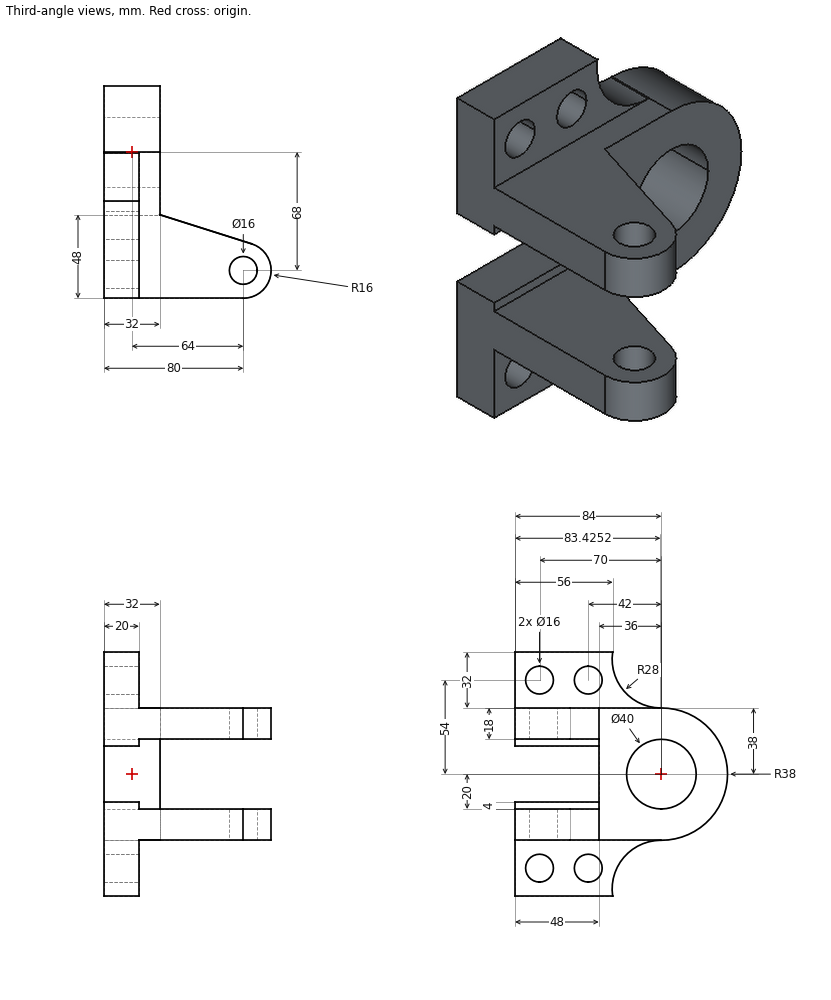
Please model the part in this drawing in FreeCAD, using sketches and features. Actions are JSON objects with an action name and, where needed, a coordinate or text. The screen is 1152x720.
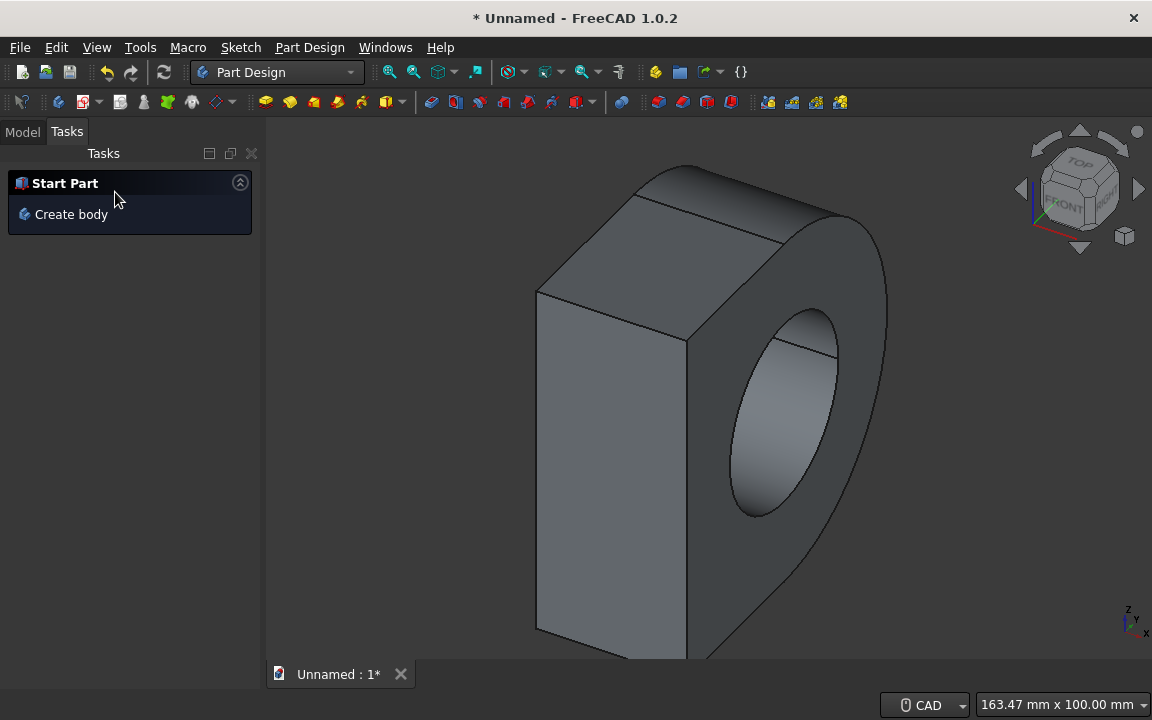
{"action": "left_click", "coordinate": [390, 72]}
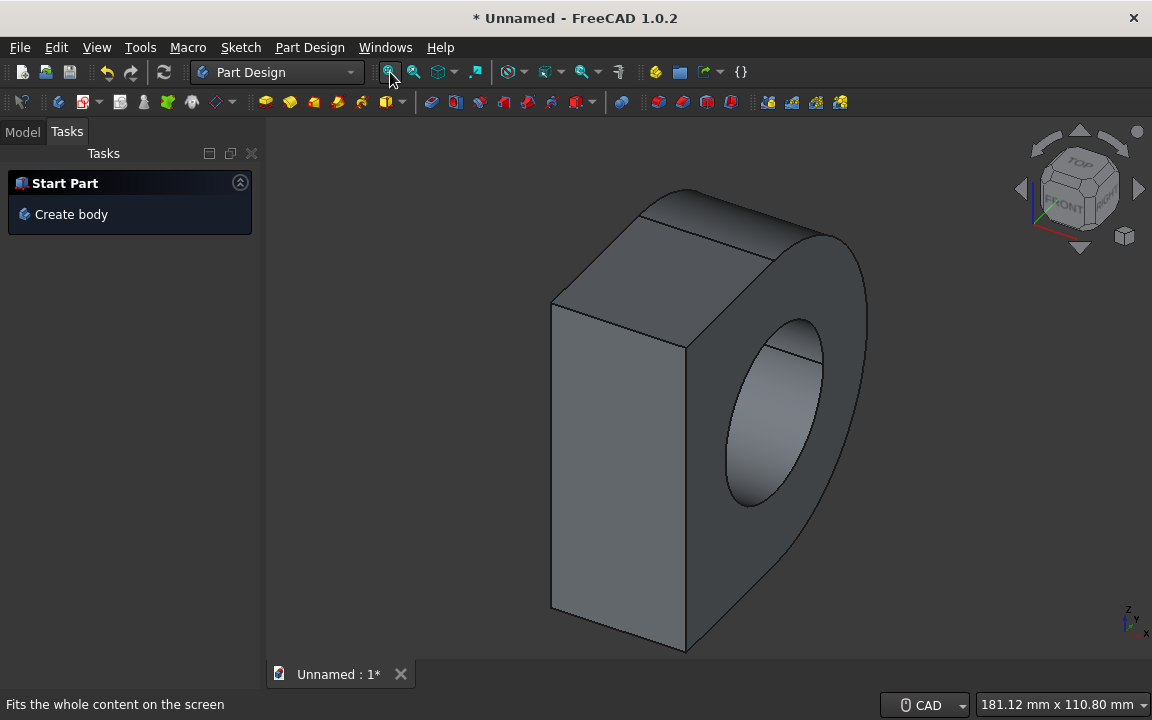
{"action": "left_click", "coordinate": [663, 281]}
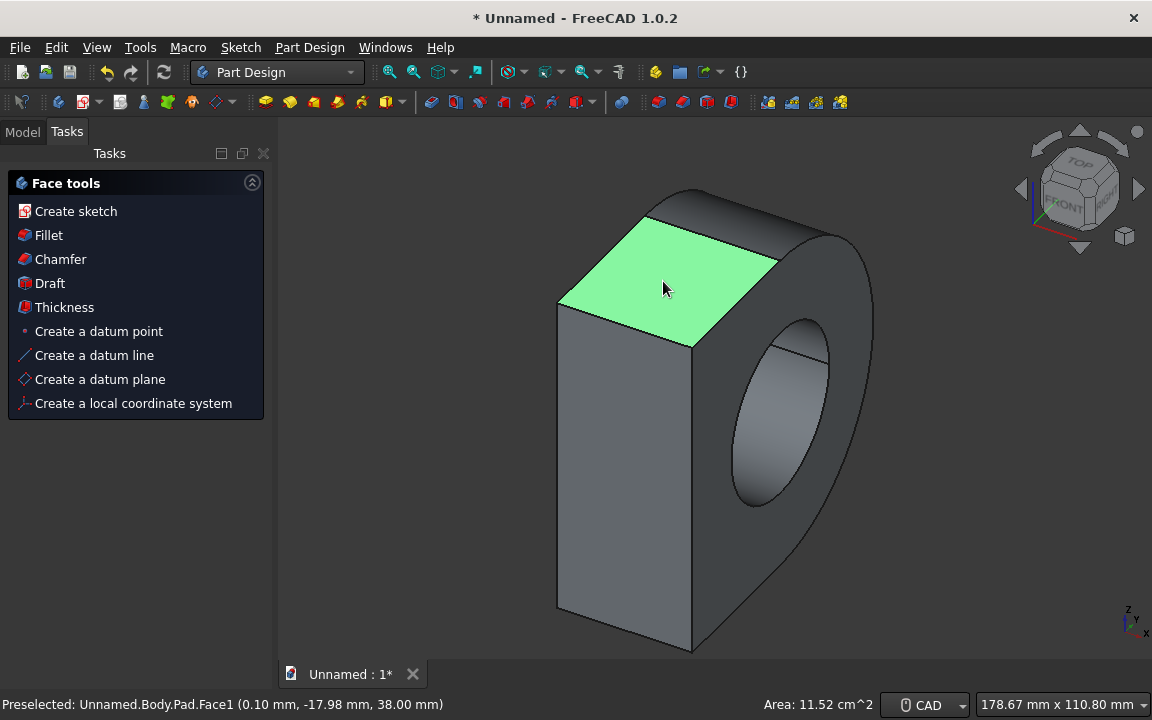
{"action": "left_click", "coordinate": [84, 102]}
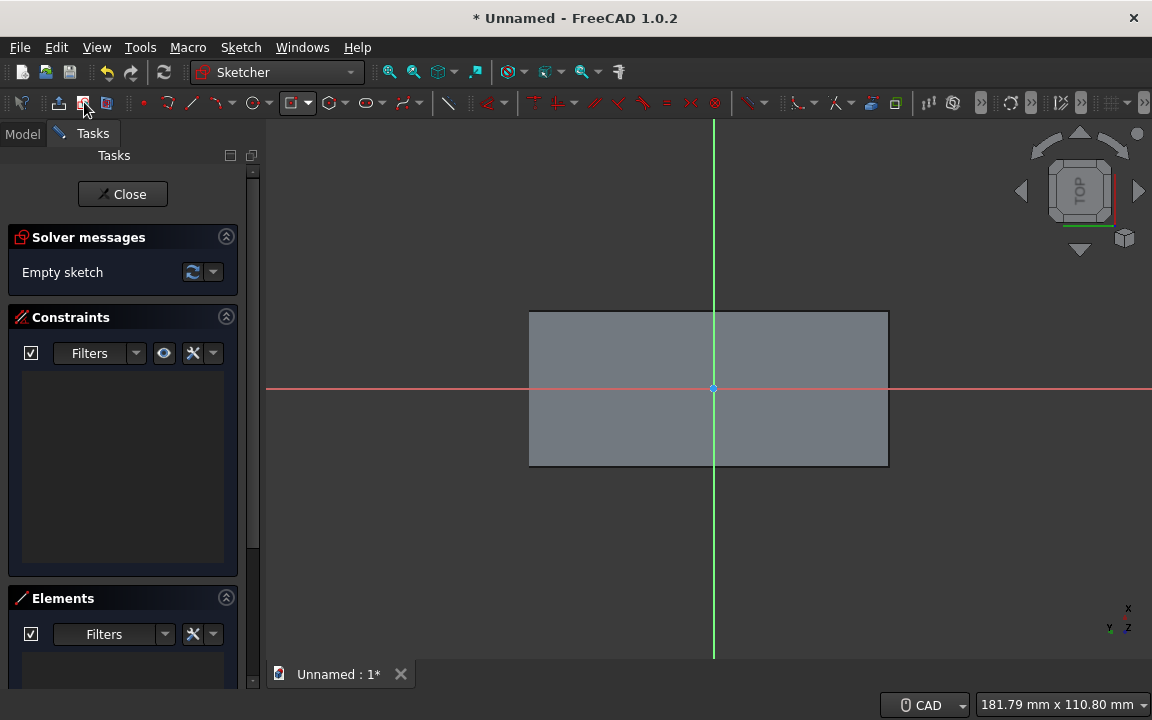
{"action": "scroll", "coordinate": [294, 631], "scroll_direction": "down", "scroll_amount": 2}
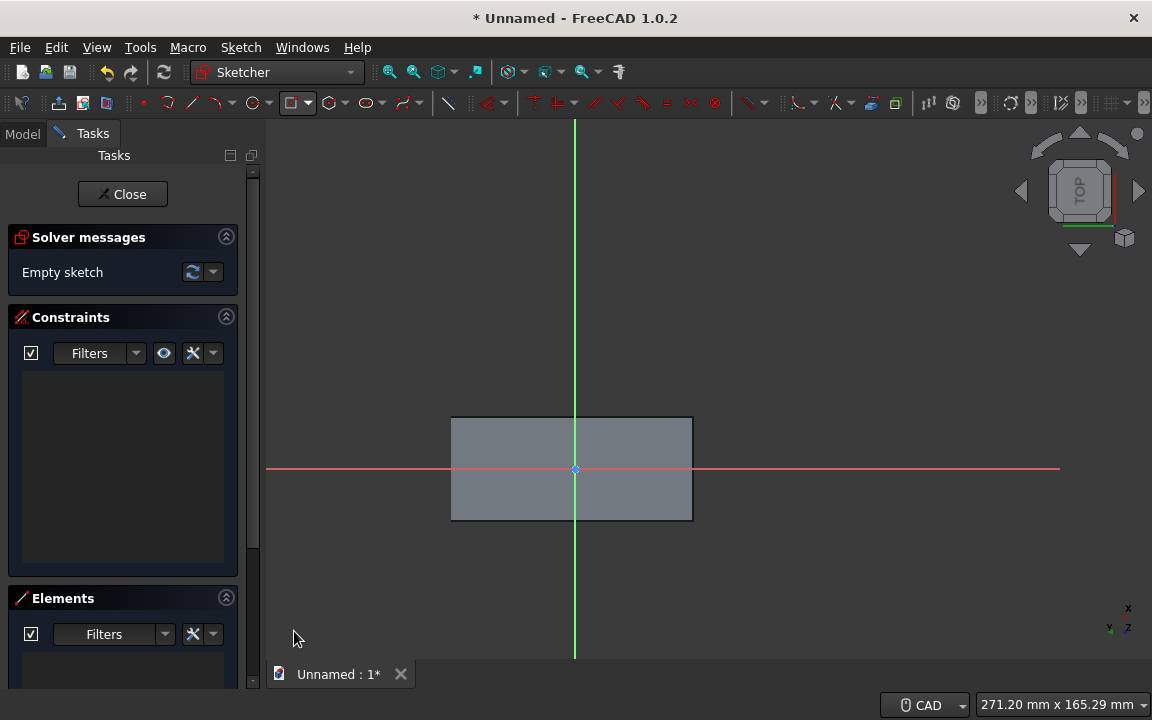
{"action": "left_click", "coordinate": [168, 104]}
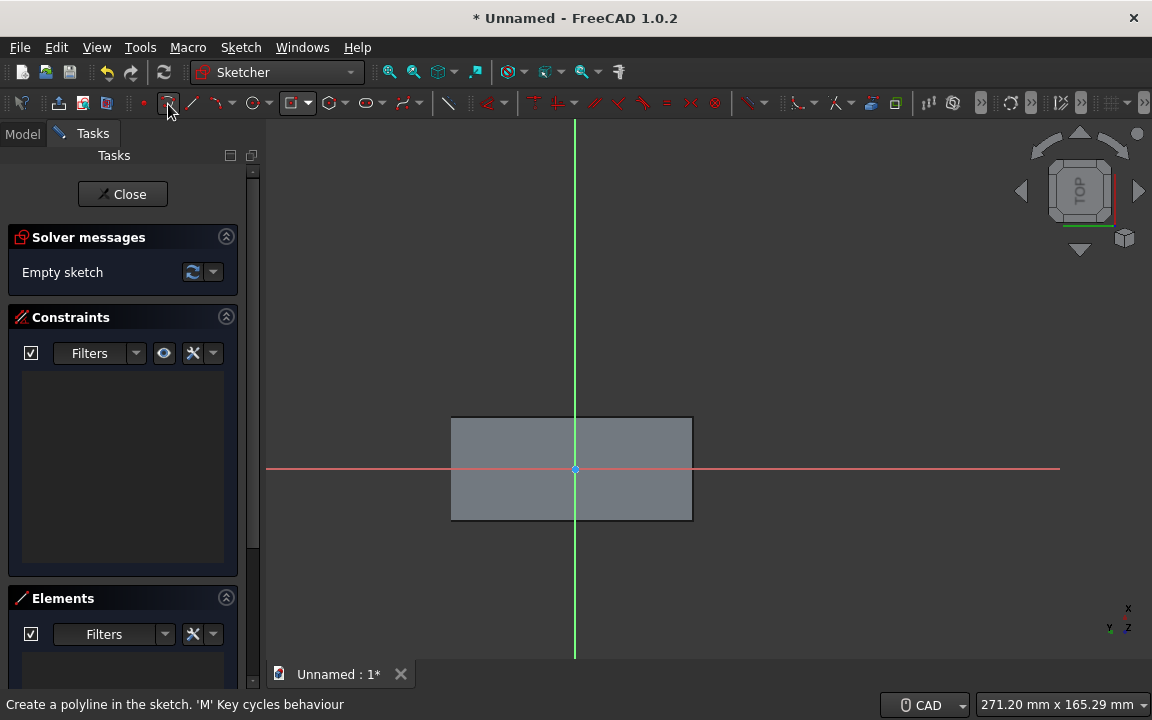
{"action": "left_click", "coordinate": [748, 244]}
{"action": "left_click", "coordinate": [693, 417]}
{"action": "left_click", "coordinate": [693, 521]}
{"action": "left_click", "coordinate": [850, 521]}
{"action": "left_click", "coordinate": [850, 260]}
{"action": "right_click", "coordinate": [850, 260]}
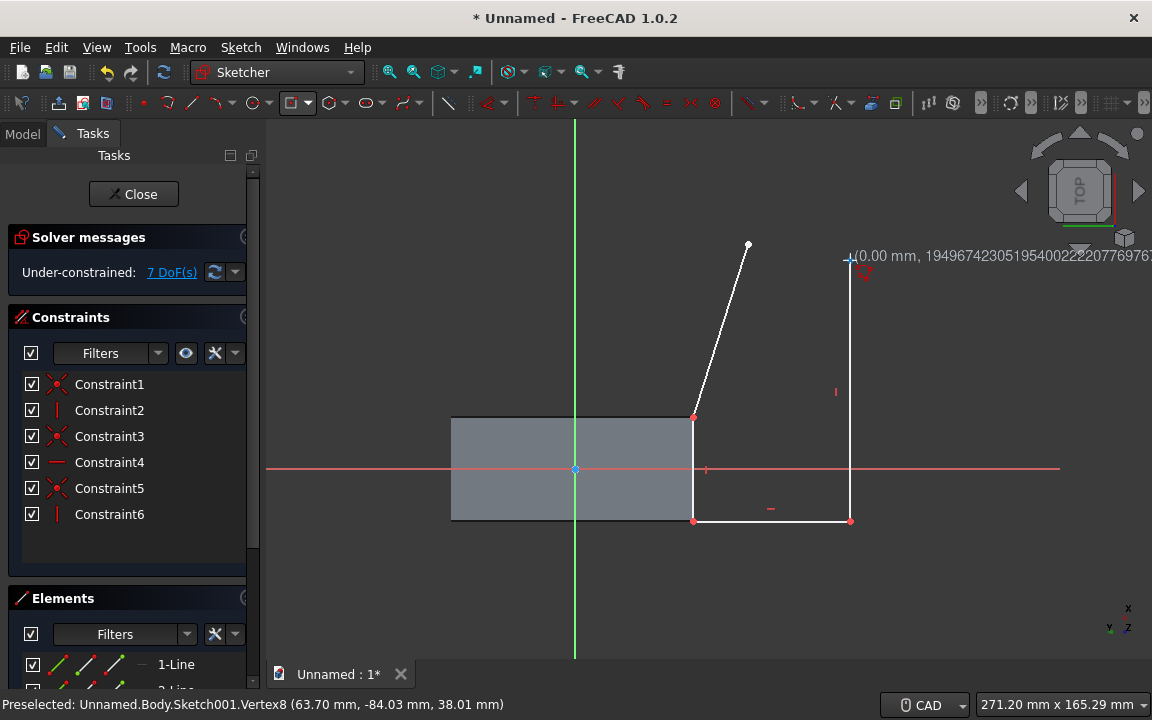
{"action": "left_click", "coordinate": [216, 104]}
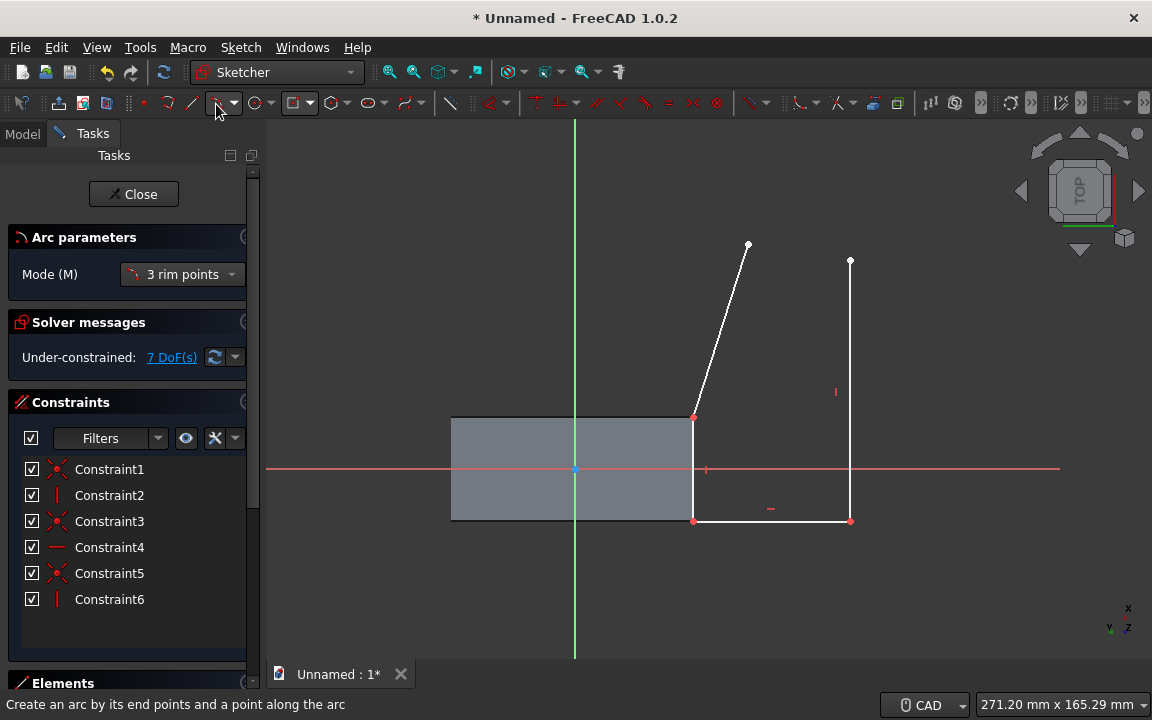
{"action": "left_click", "coordinate": [850, 261]}
{"action": "left_click", "coordinate": [748, 245]}
{"action": "left_click", "coordinate": [806, 208]}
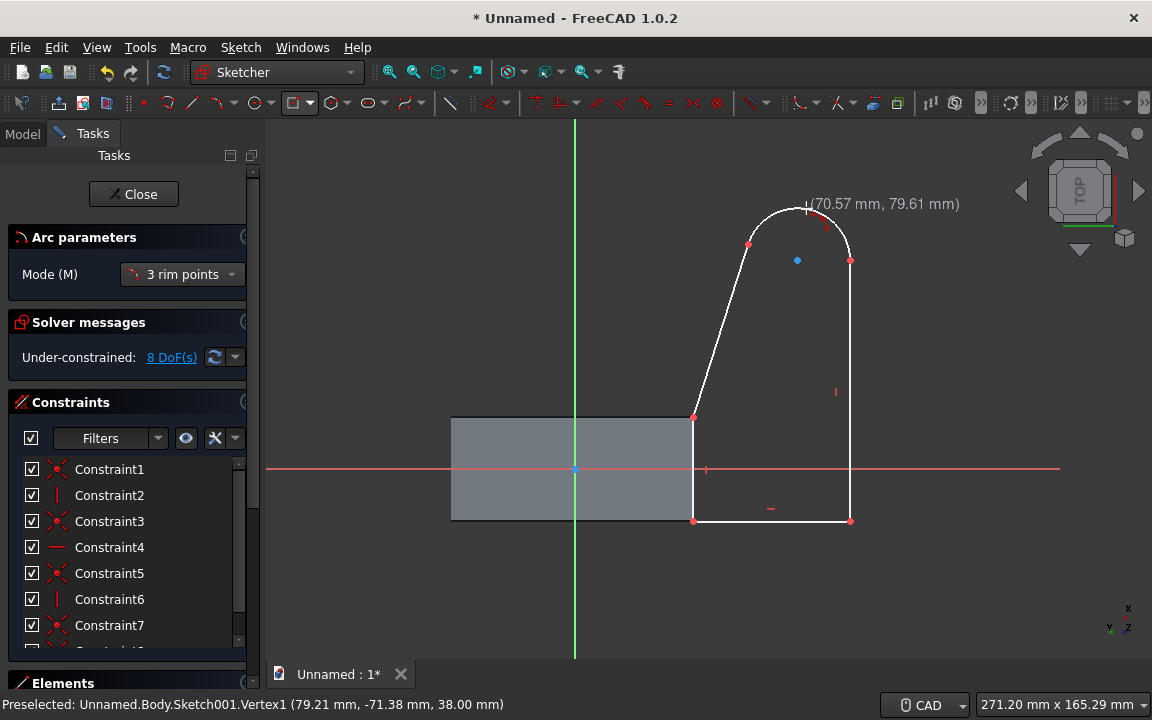
{"action": "left_click", "coordinate": [256, 104]}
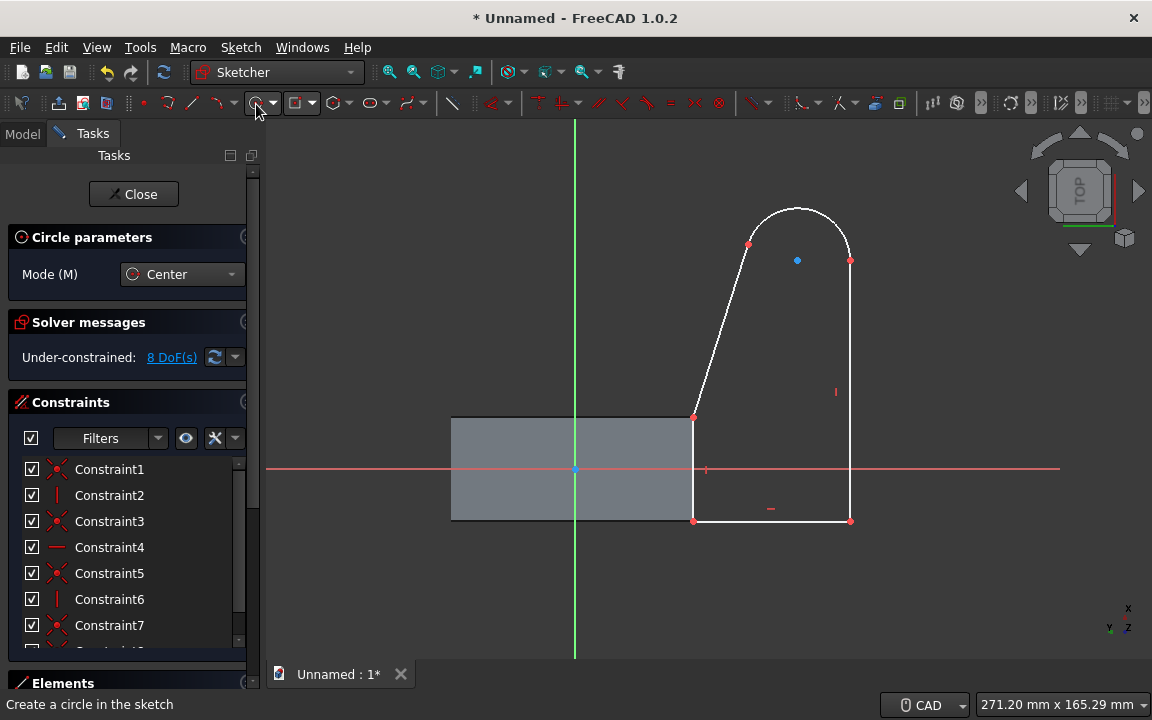
{"action": "left_click", "coordinate": [798, 260]}
{"action": "left_click", "coordinate": [816, 242]}
{"action": "key", "text": "Escape"}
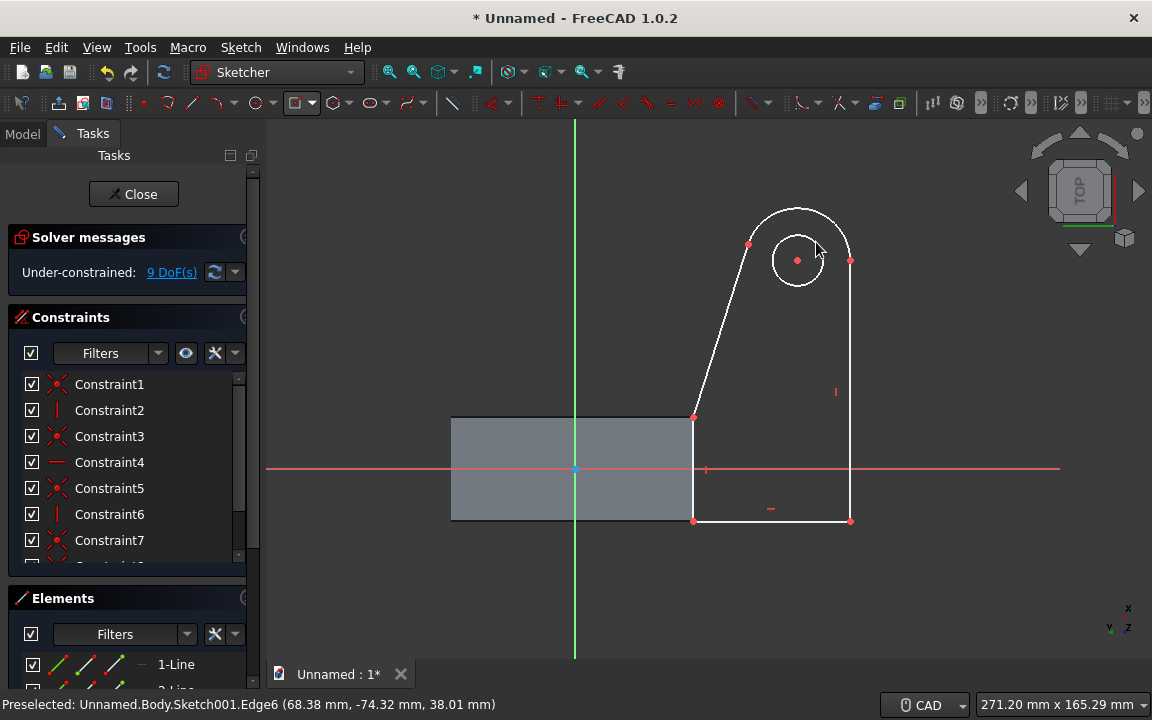
{"action": "left_click", "coordinate": [731, 297]}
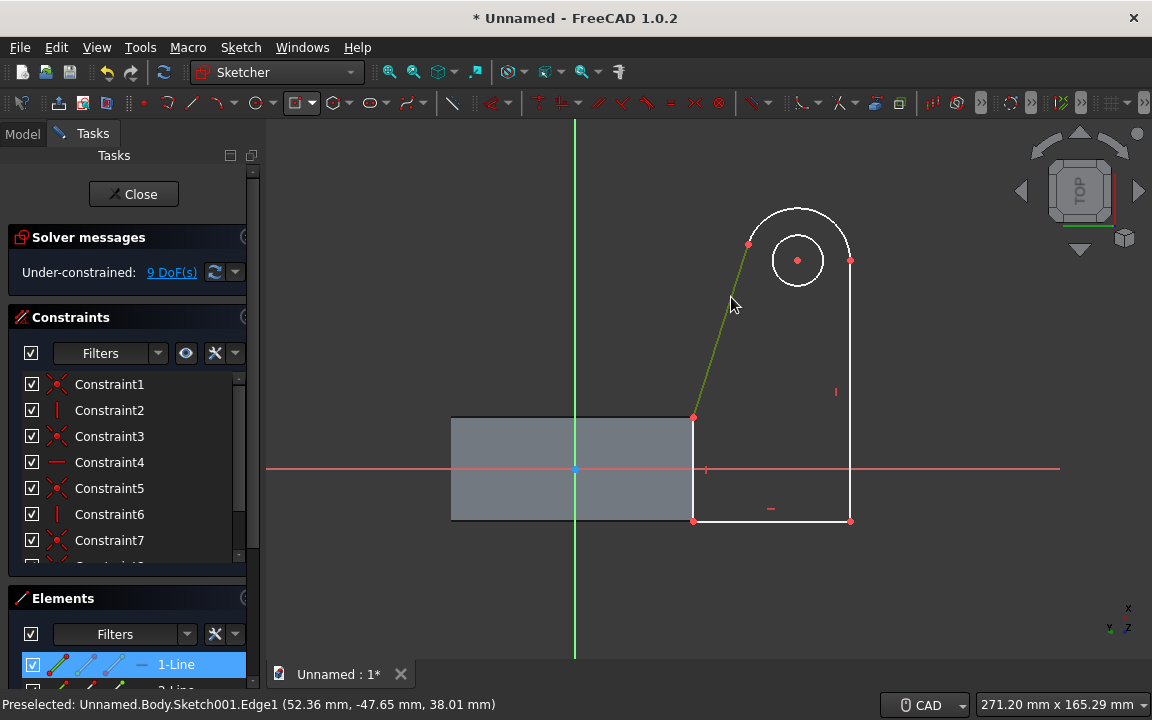
{"action": "left_click", "coordinate": [832, 221]}